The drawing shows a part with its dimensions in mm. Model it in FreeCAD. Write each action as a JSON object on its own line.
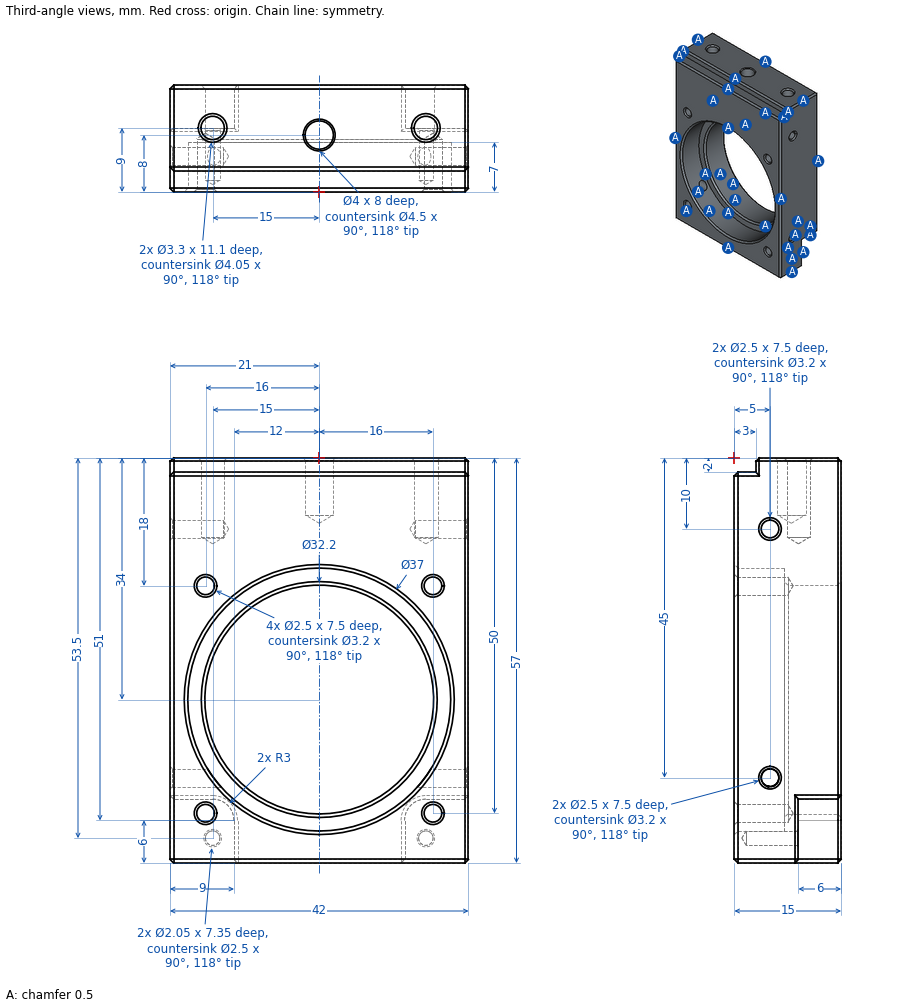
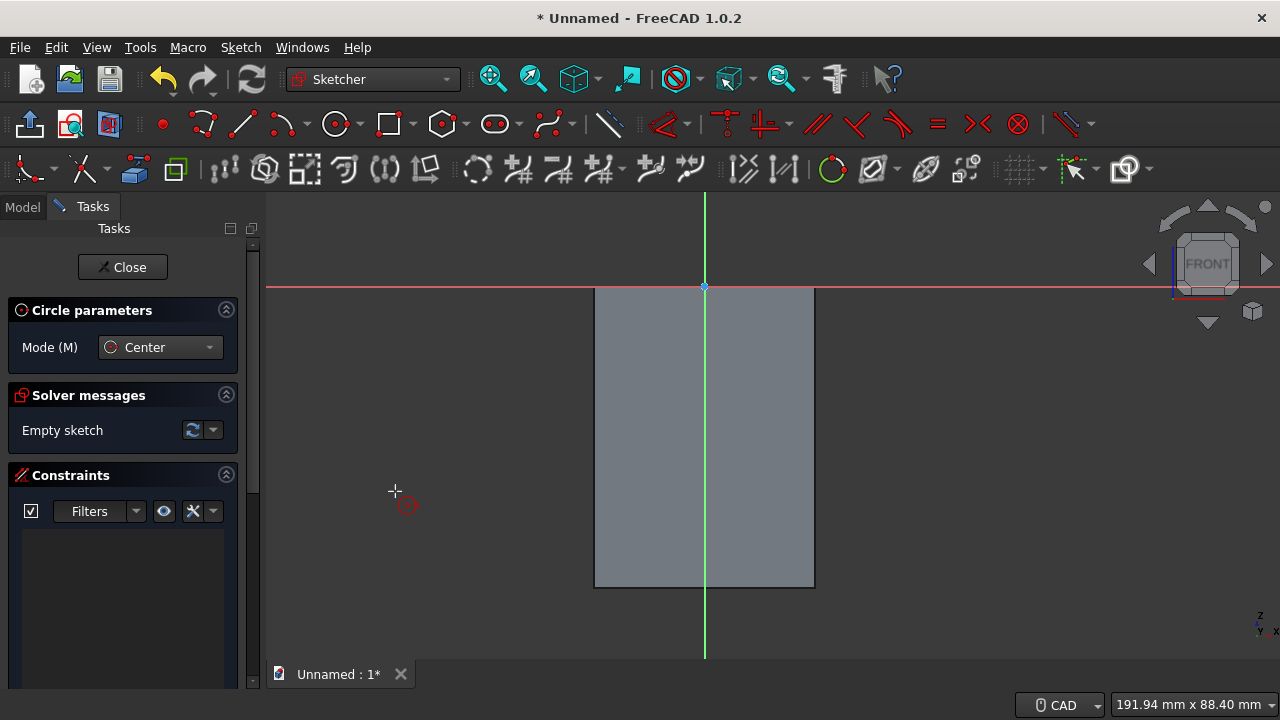
{"action": "left_click", "coordinate": [705, 467]}
{"action": "mouse_move", "coordinate": [774, 397]}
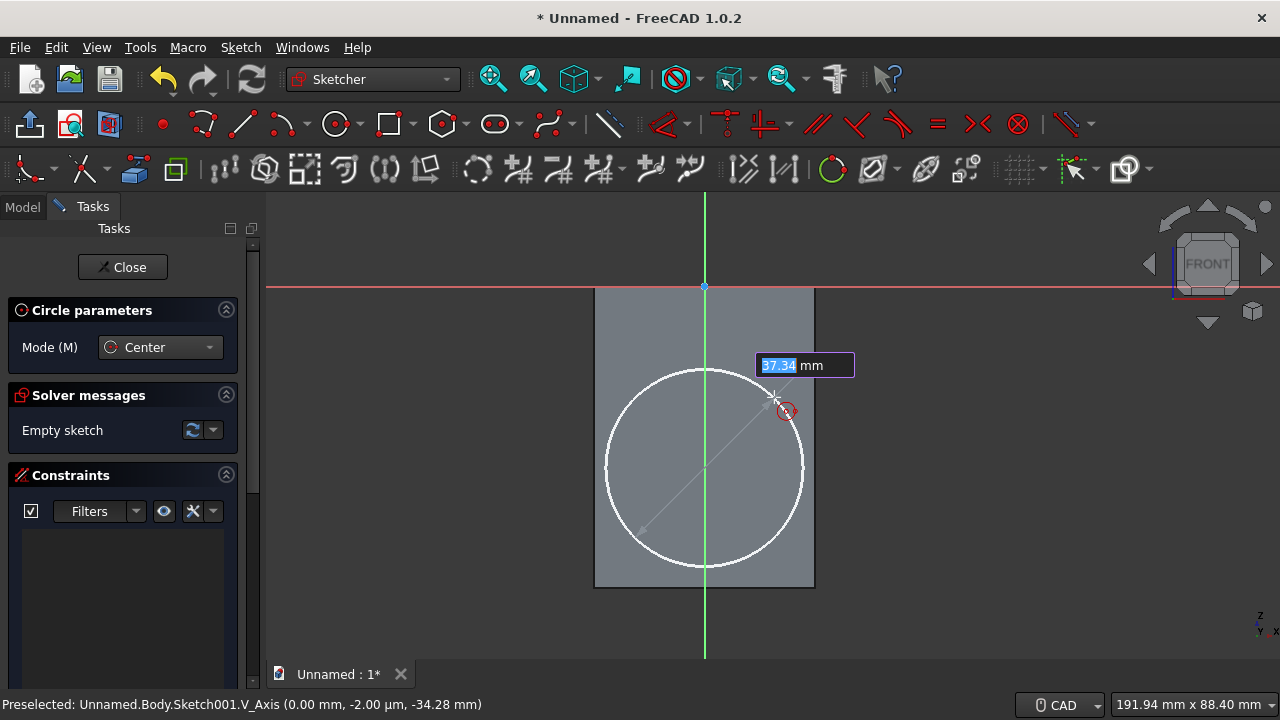
{"action": "type", "text": "37"}
{"action": "key", "text": "Return"}
{"action": "key", "text": "Escape"}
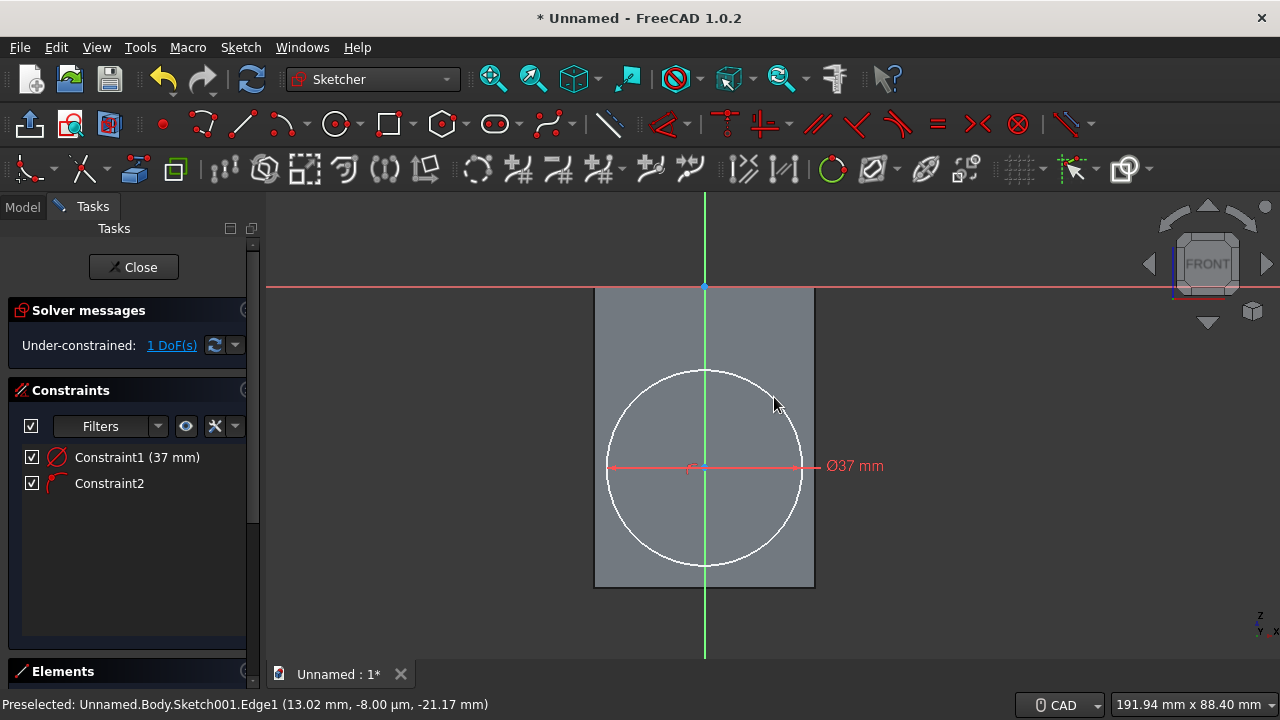
{"action": "key", "text": "d"}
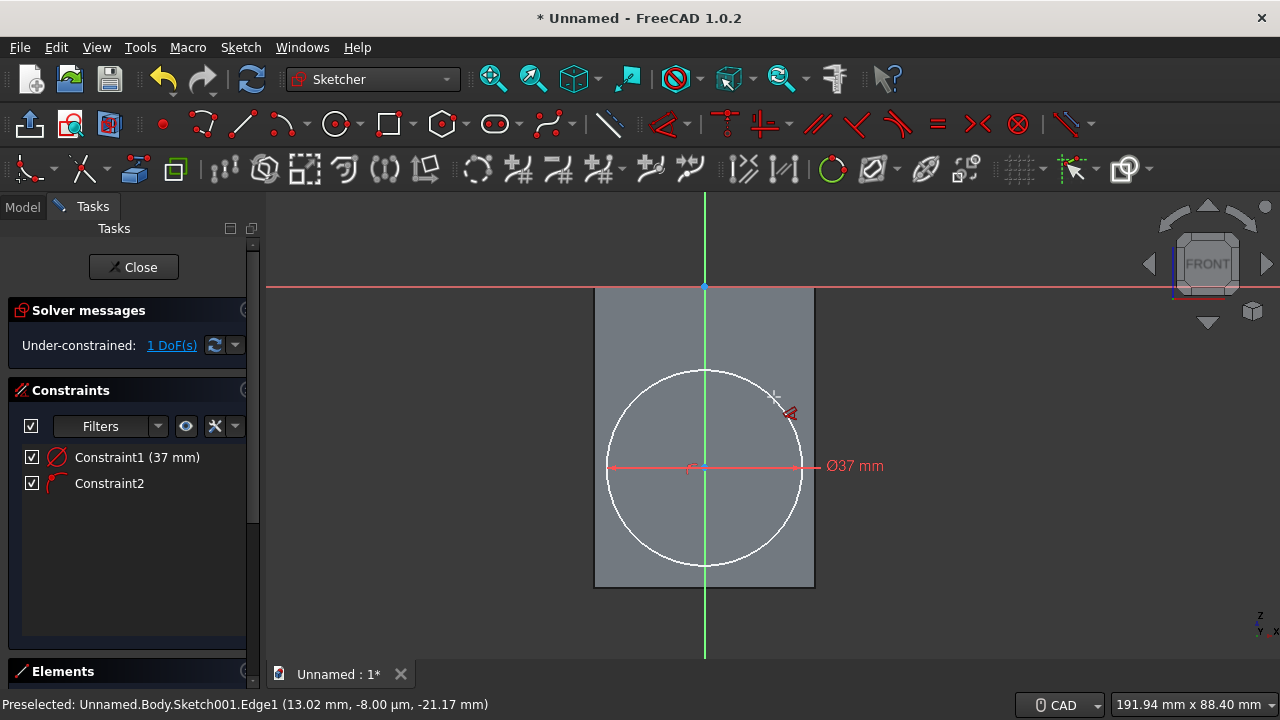
{"action": "left_click", "coordinate": [705, 468]}
{"action": "left_click", "coordinate": [739, 336]}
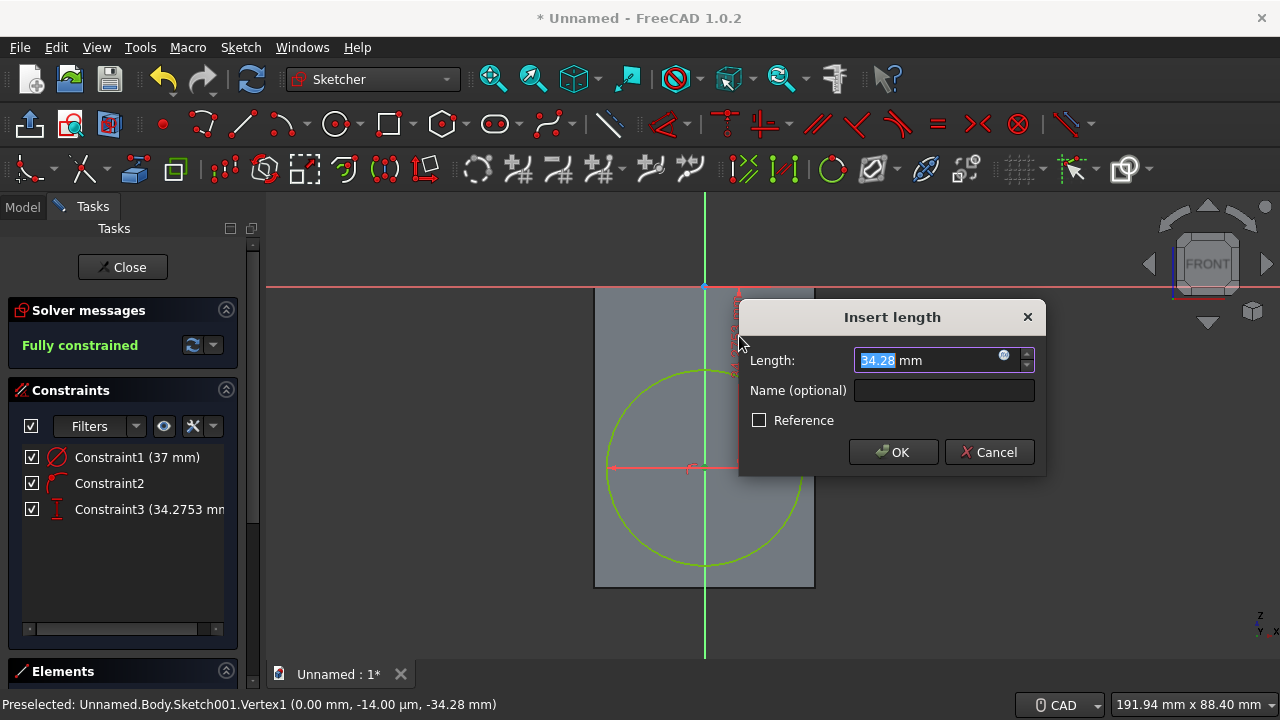
{"action": "type", "text": "34"}
{"action": "key", "text": "Return"}
{"action": "key", "text": "Escape"}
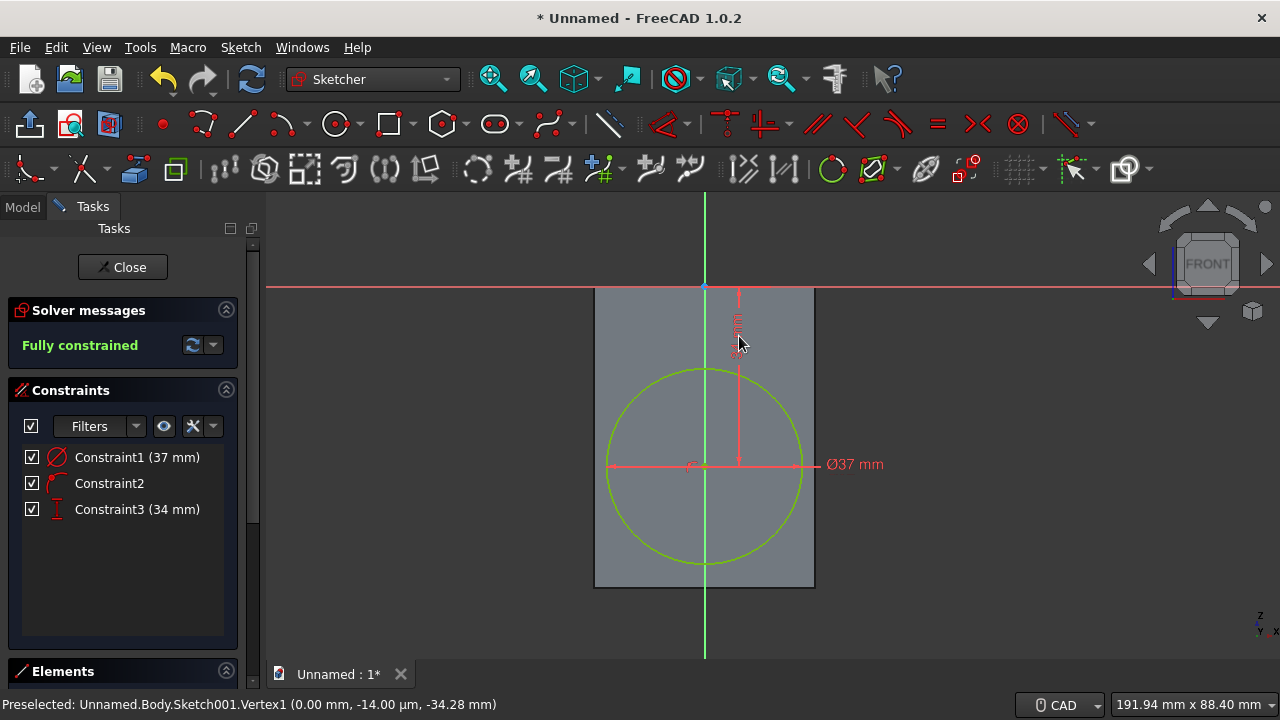
{"action": "left_click", "coordinate": [123, 267]}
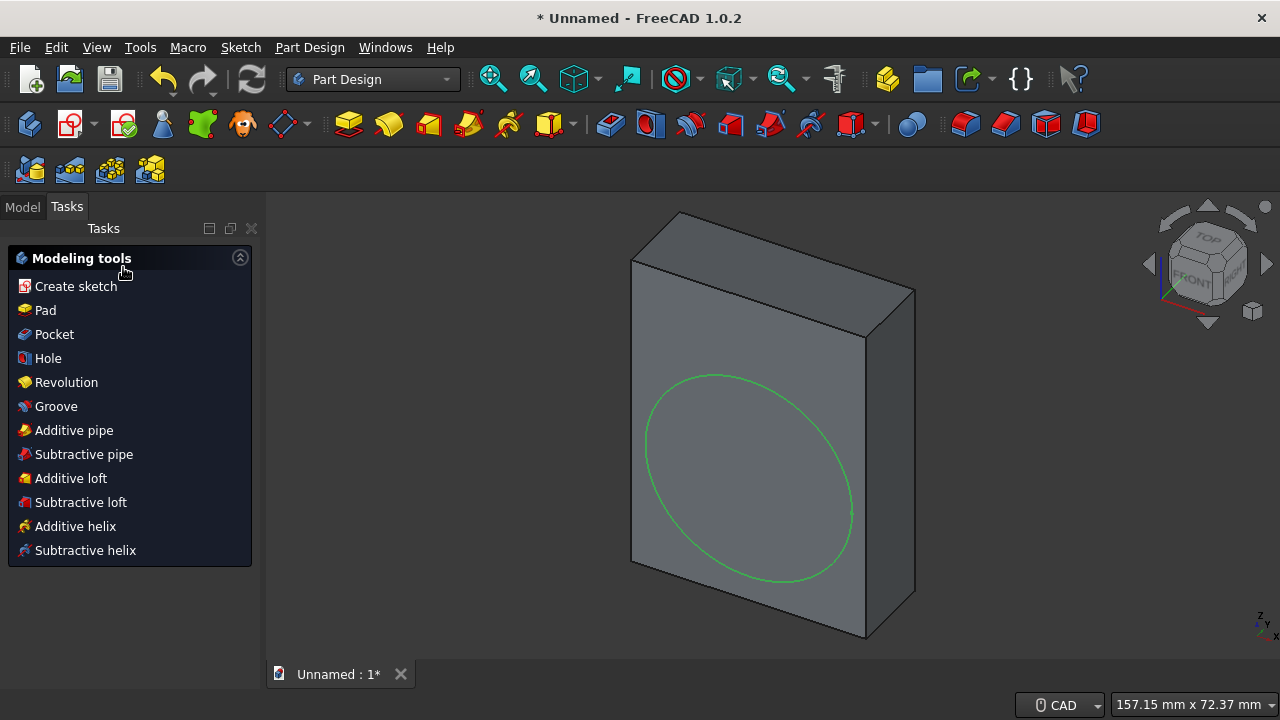
{"action": "left_click", "coordinate": [612, 124]}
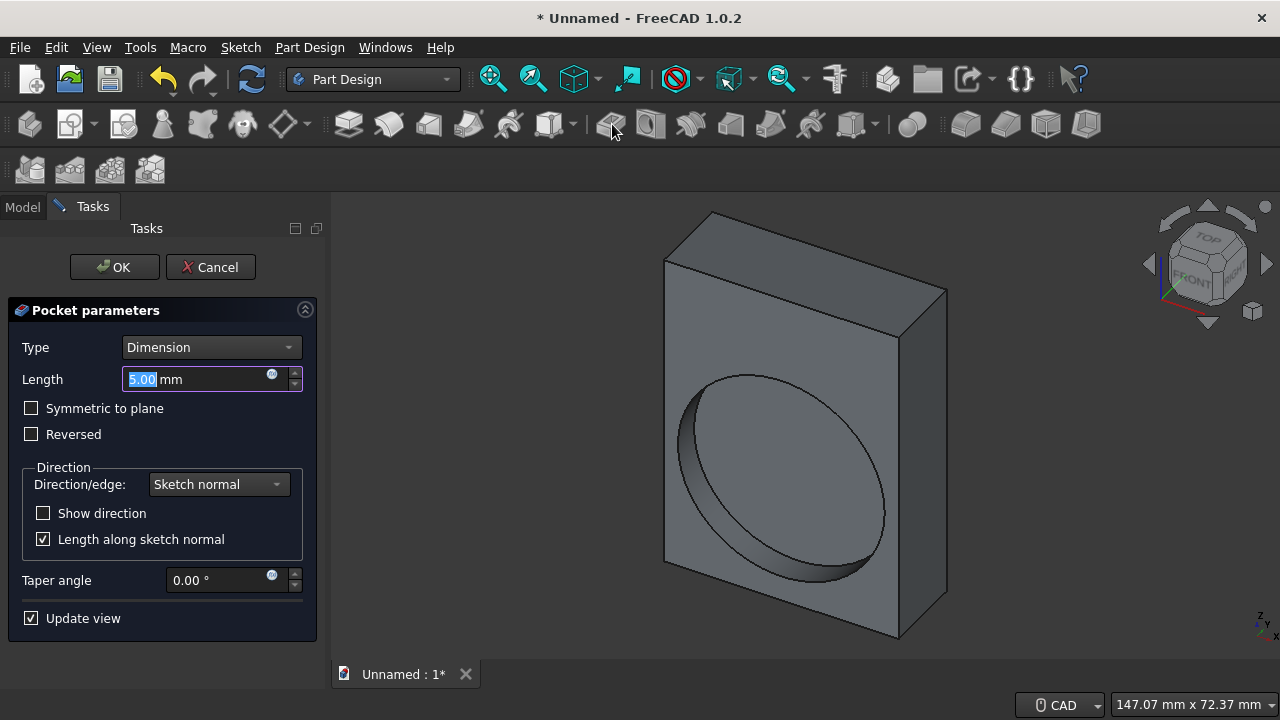
{"action": "type", "text": "7"}
{"action": "key", "text": "Tab"}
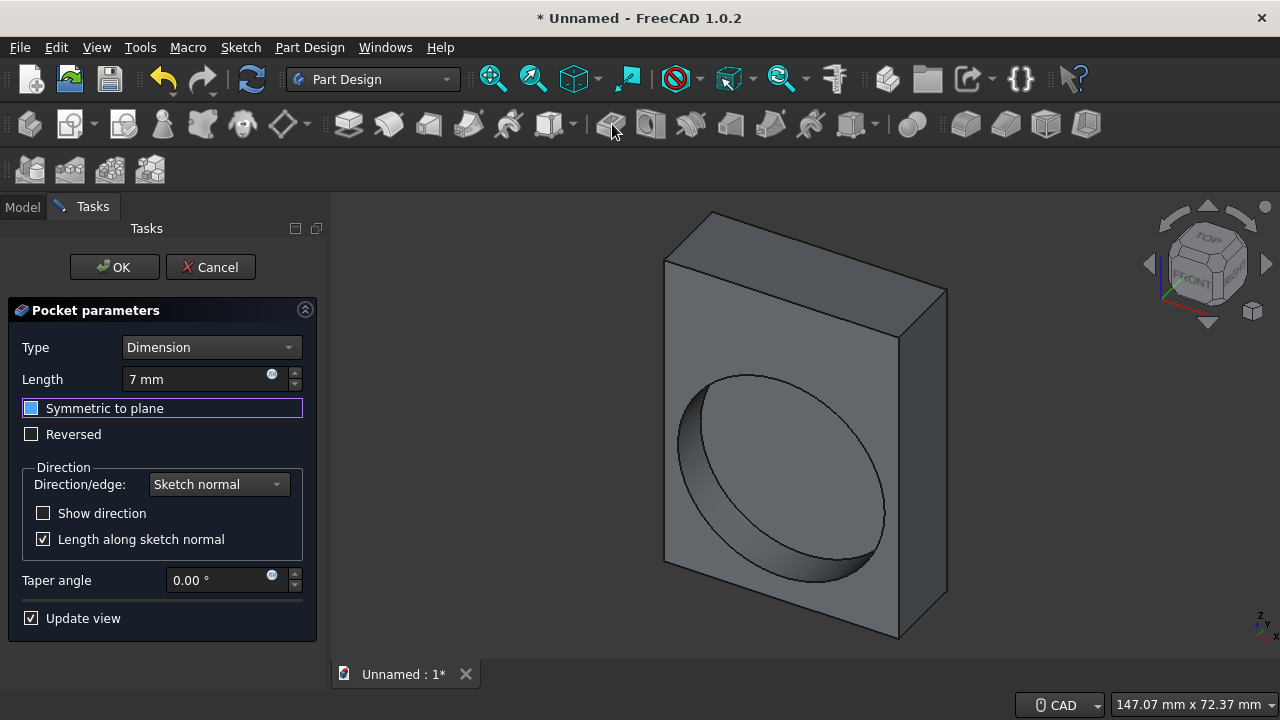
{"action": "left_click", "coordinate": [115, 267]}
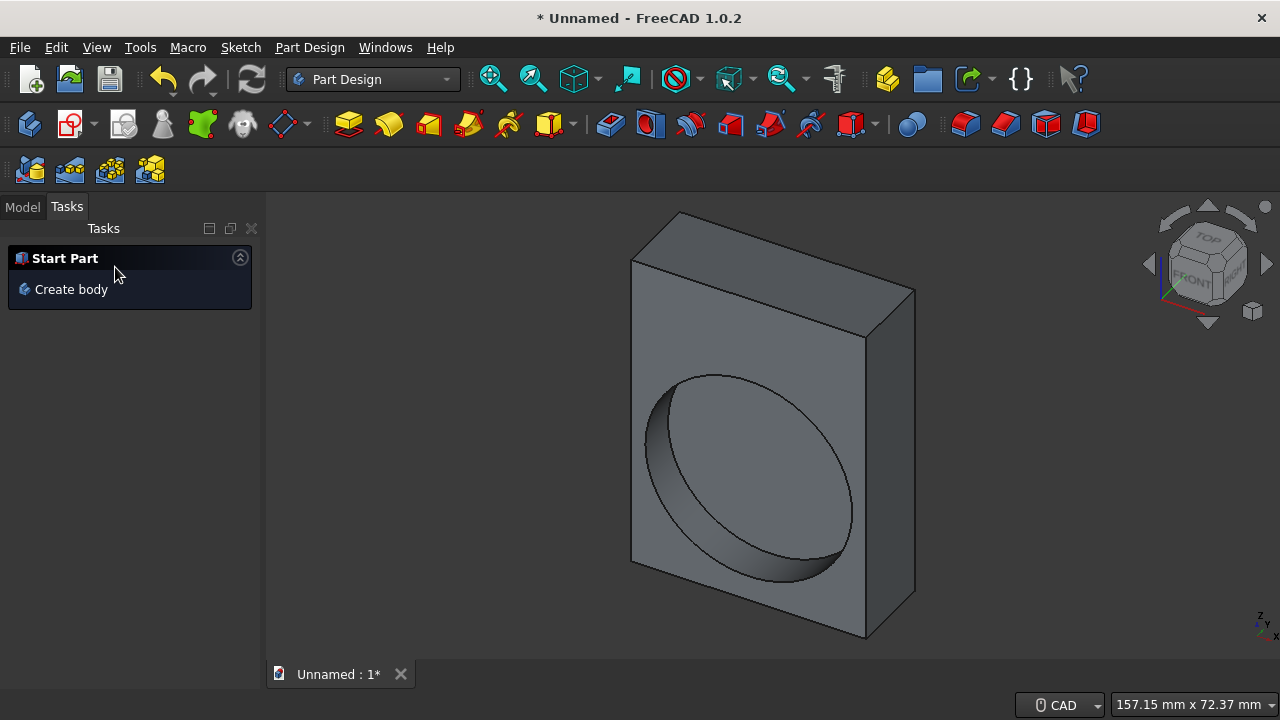
{"action": "left_click", "coordinate": [771, 455]}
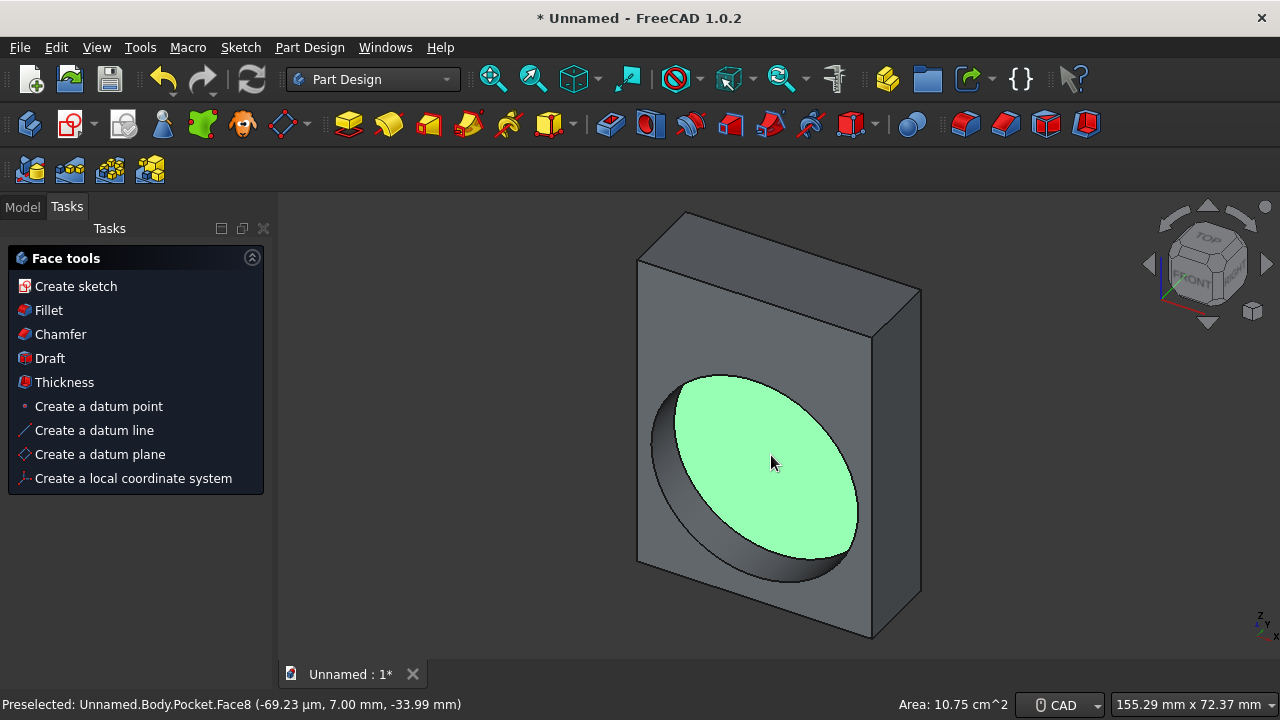
{"action": "left_click", "coordinate": [70, 124]}